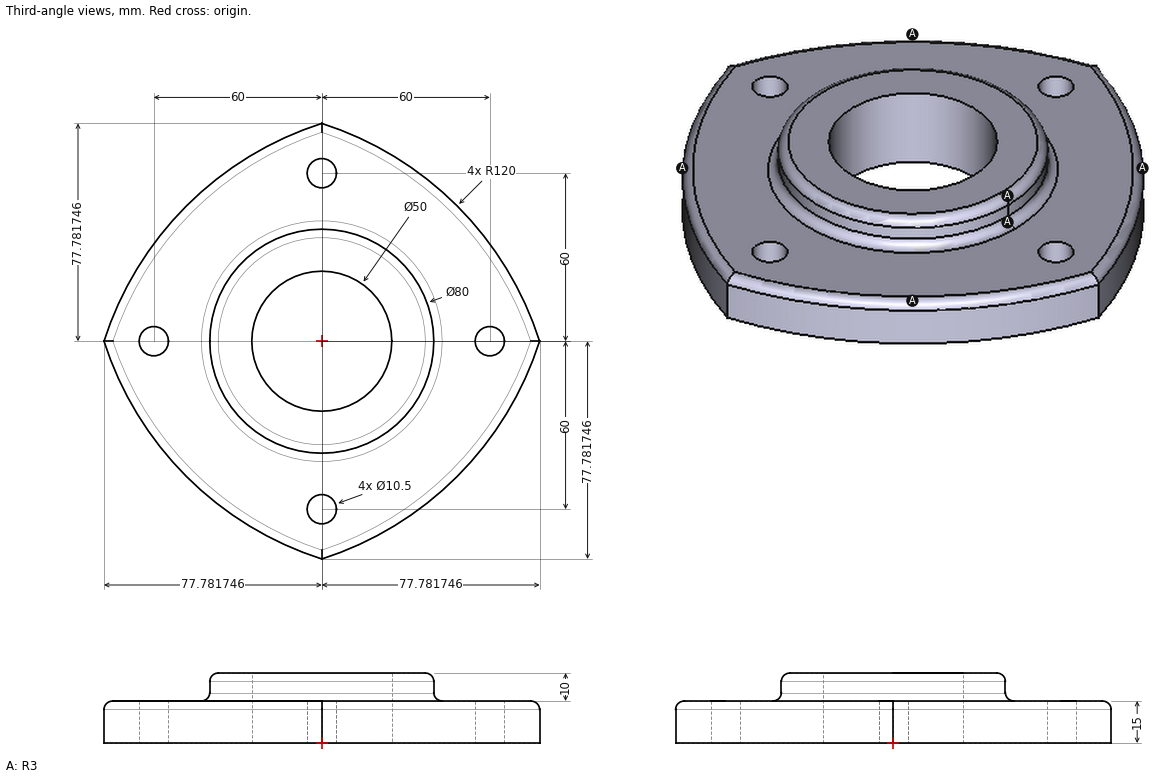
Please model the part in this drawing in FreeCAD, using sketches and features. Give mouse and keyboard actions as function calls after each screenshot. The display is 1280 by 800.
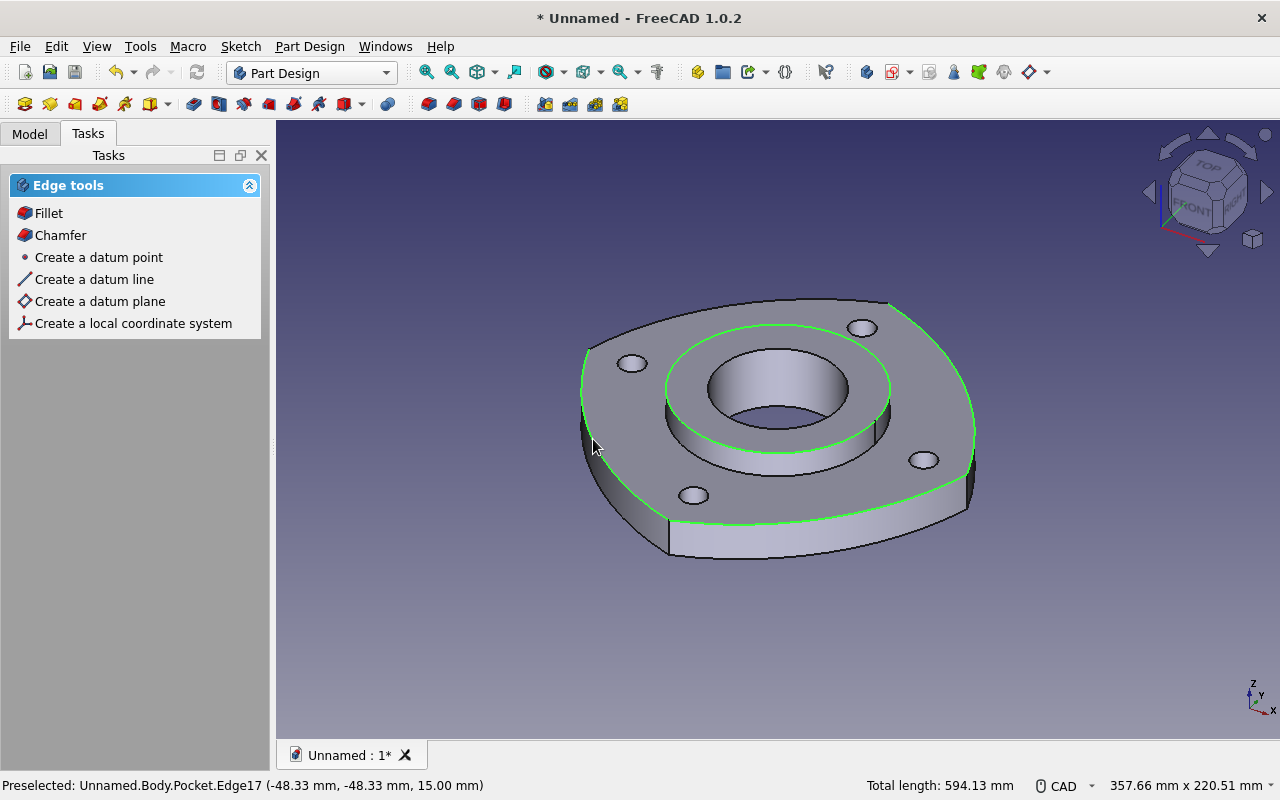
key(0)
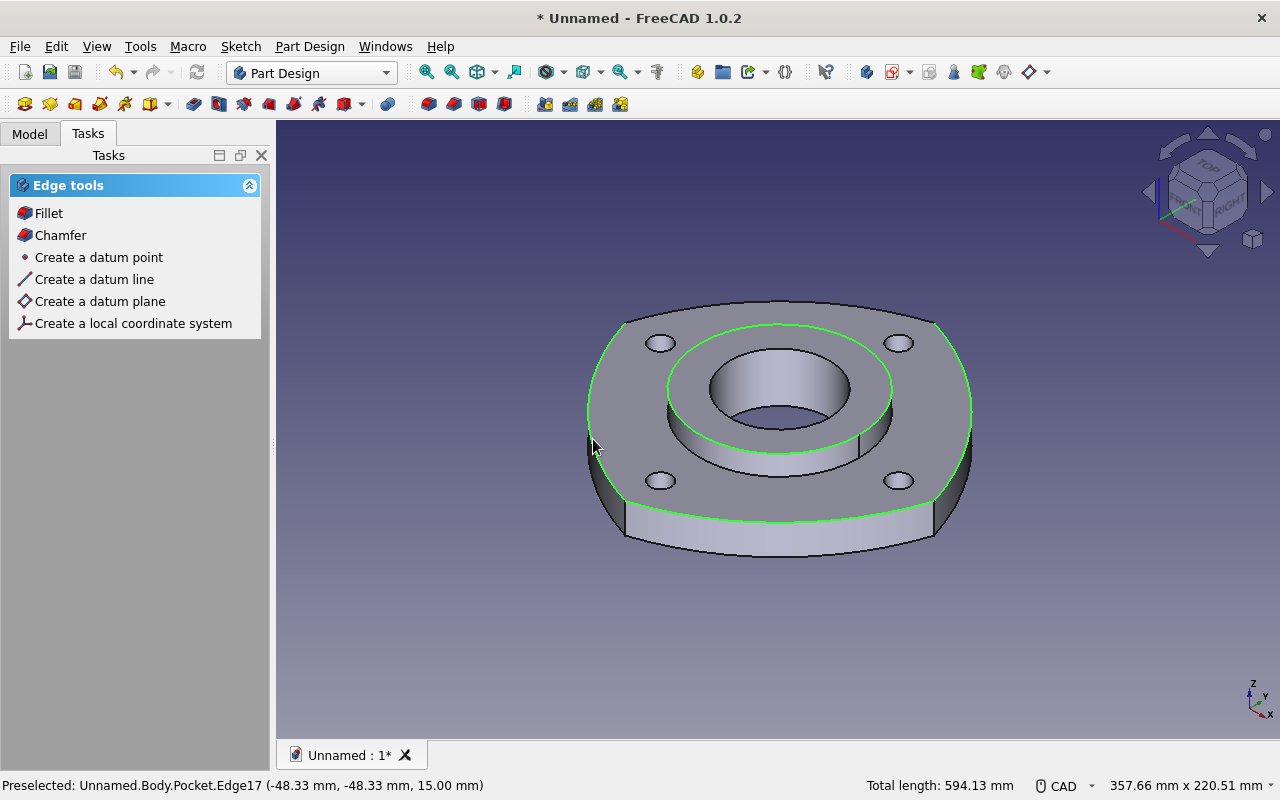
key(2)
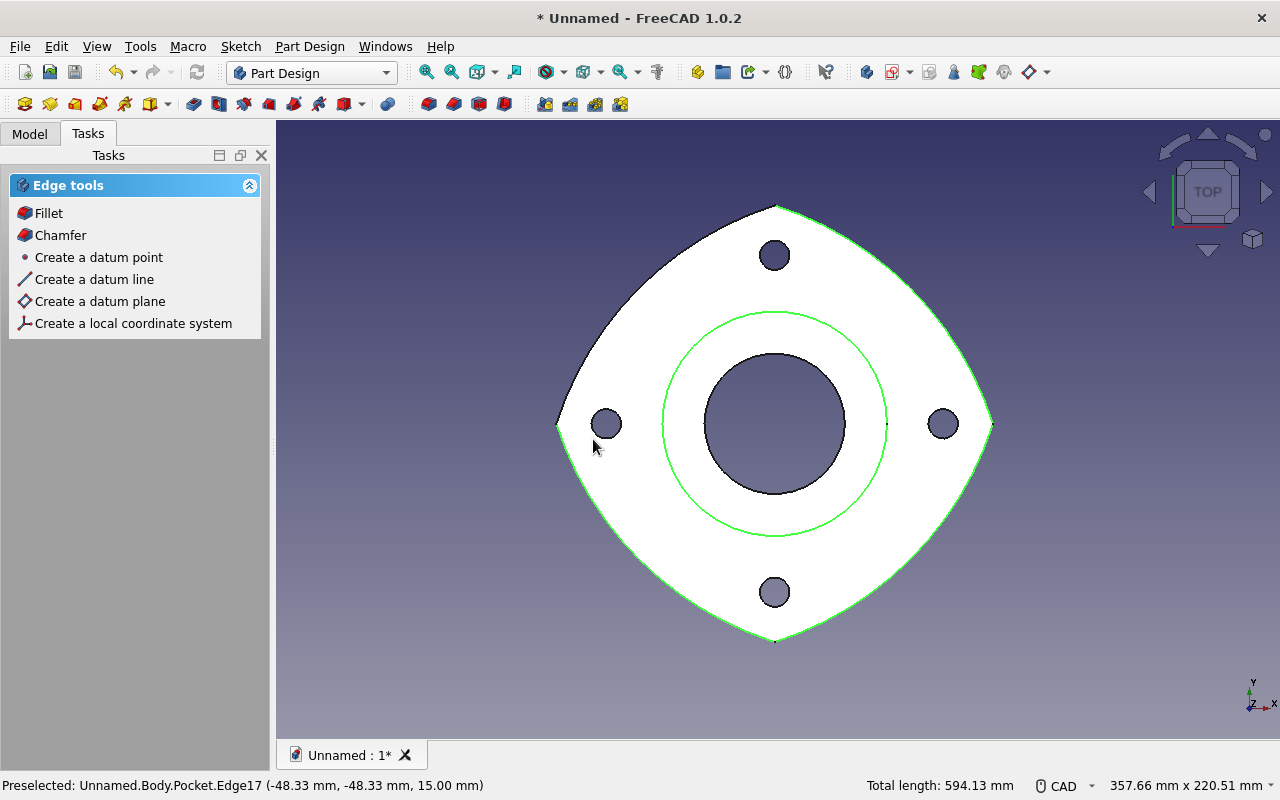
click(639, 287, ctrl)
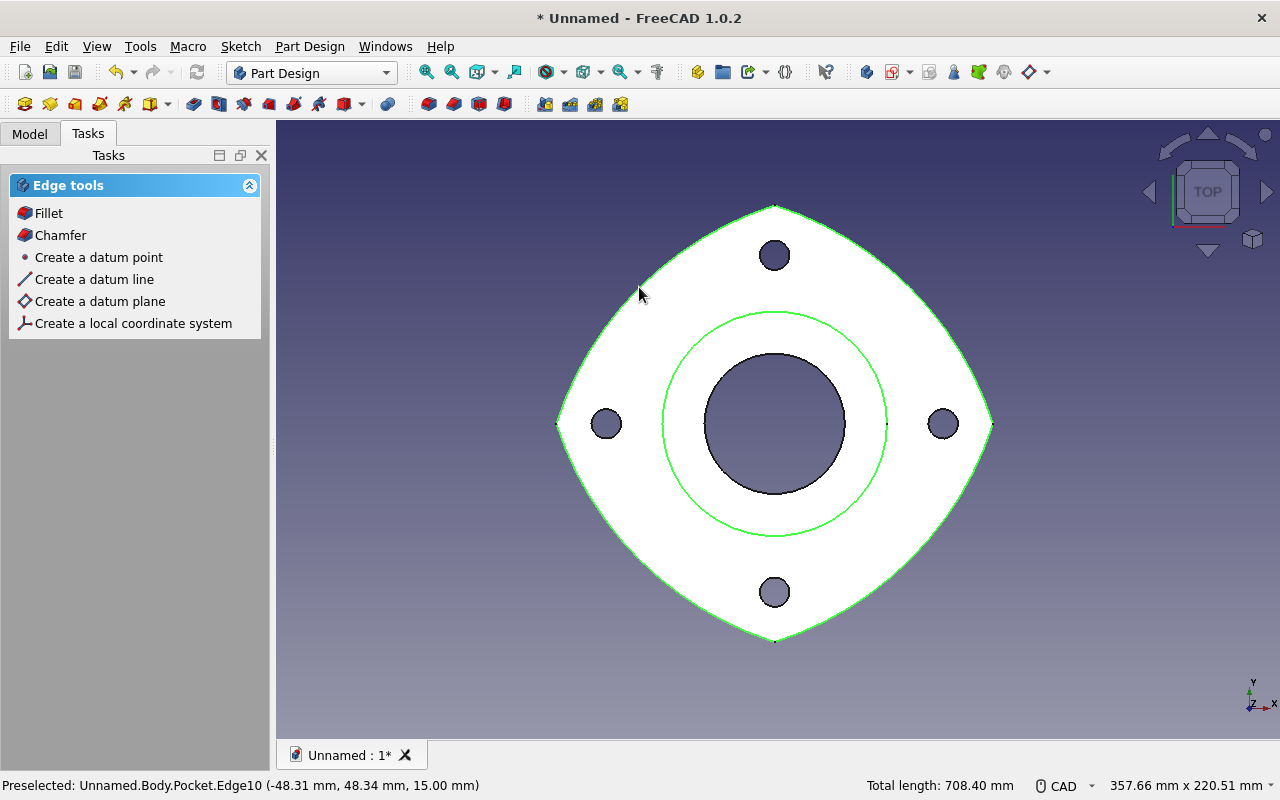
key(1)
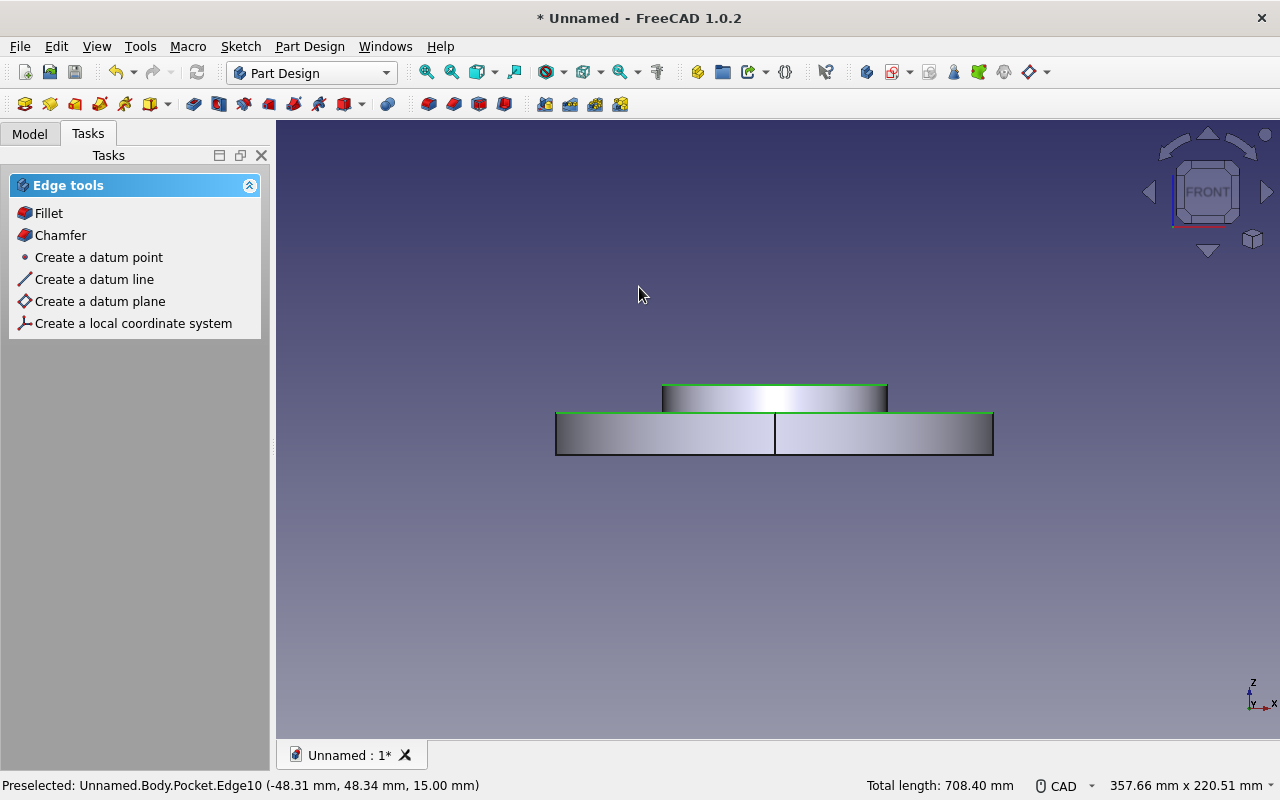
key(v)
key(f)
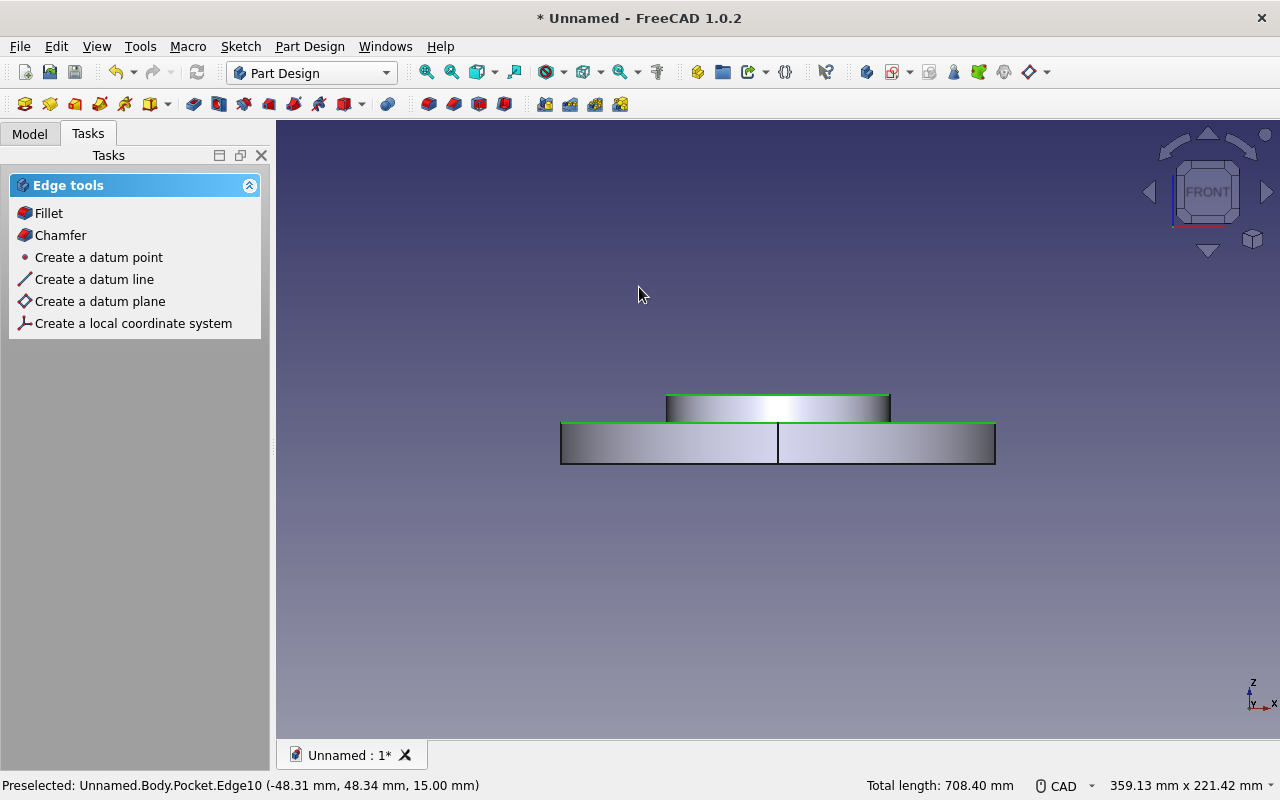
key(3)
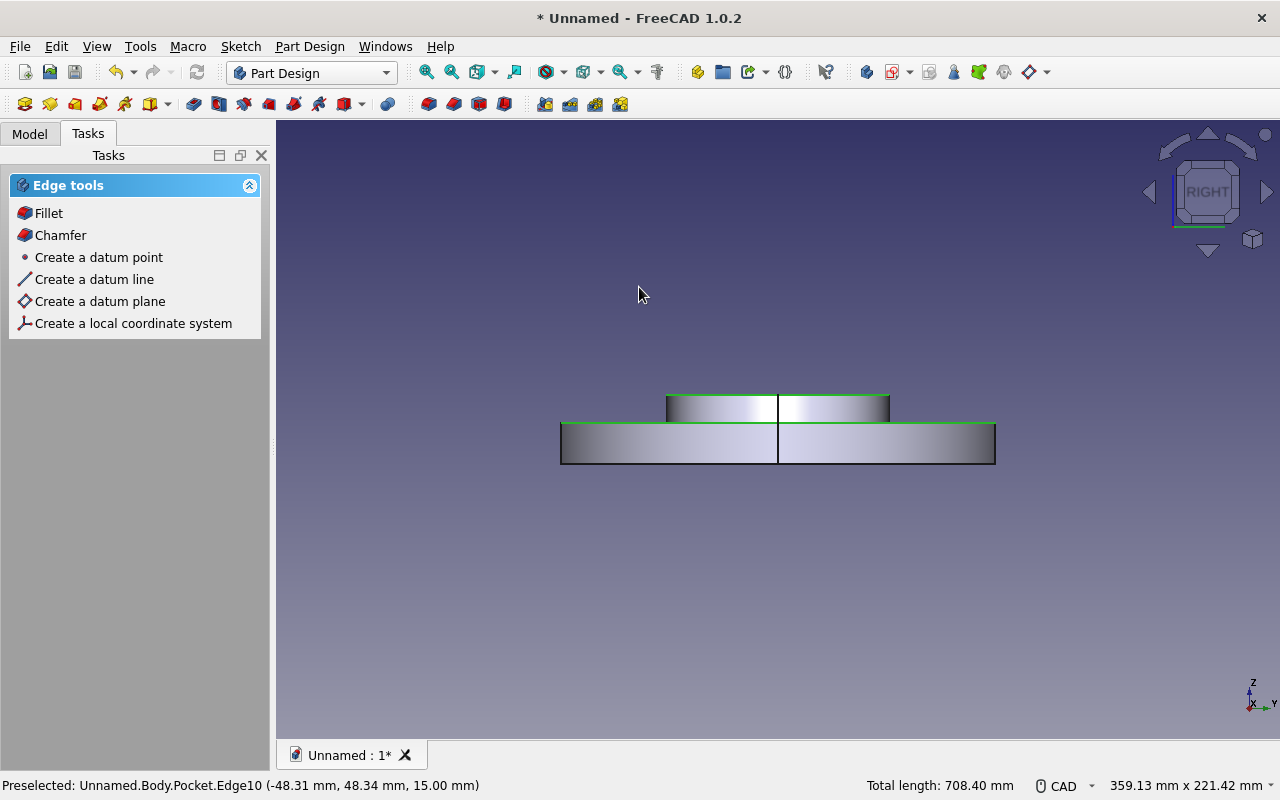
key(v)
key(f)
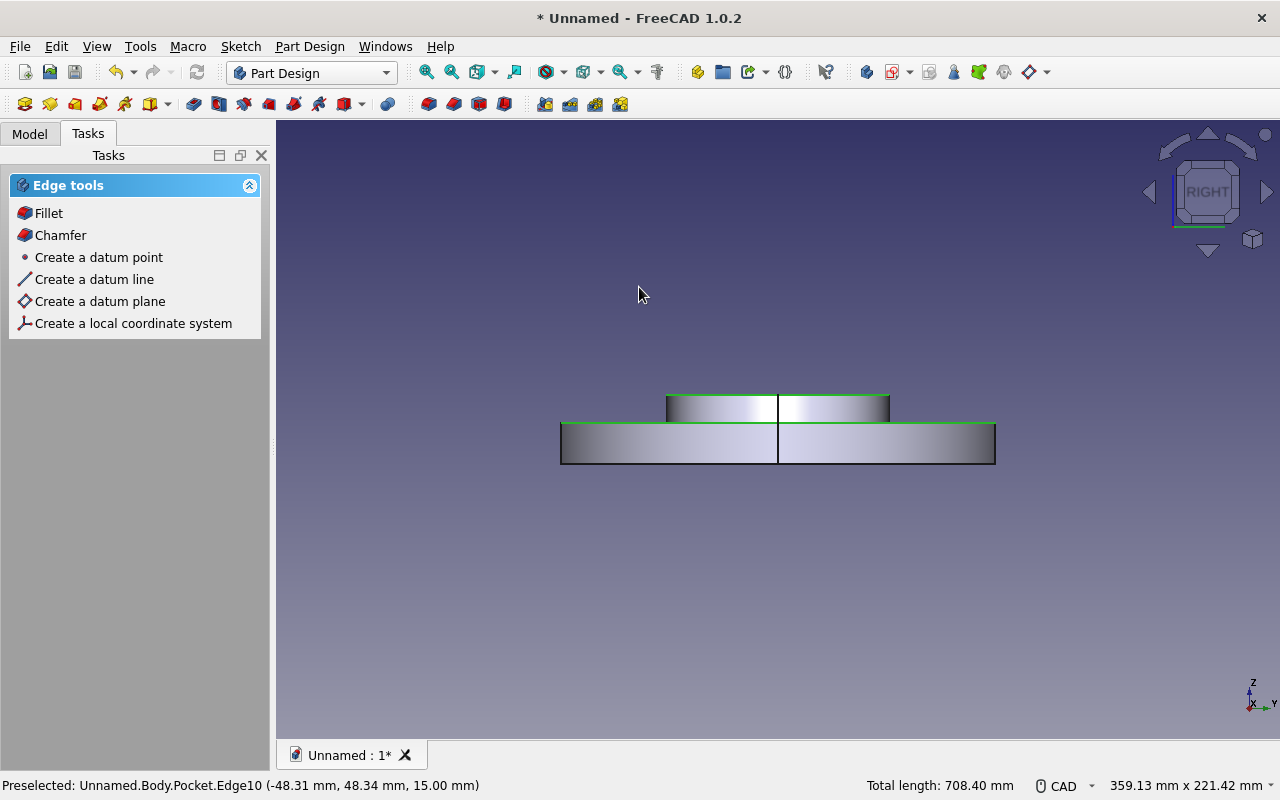
key(5)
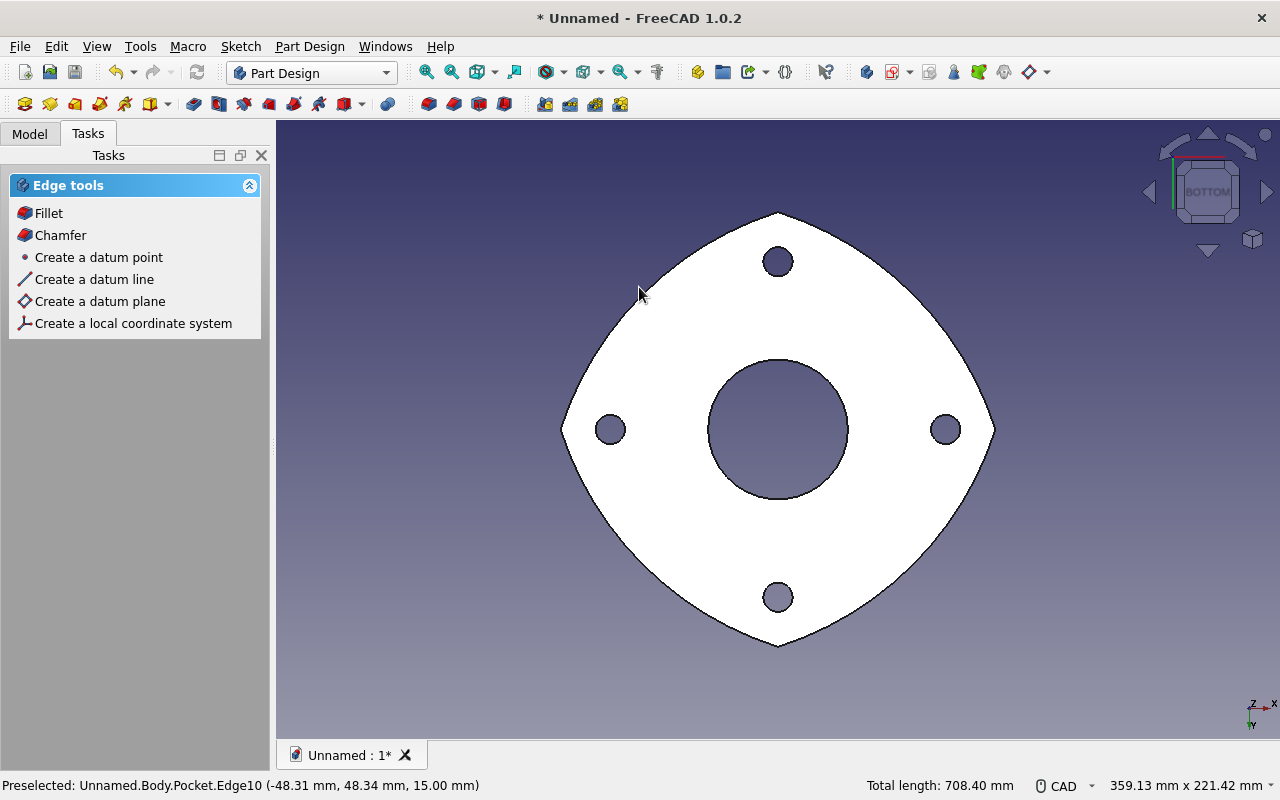
key(4)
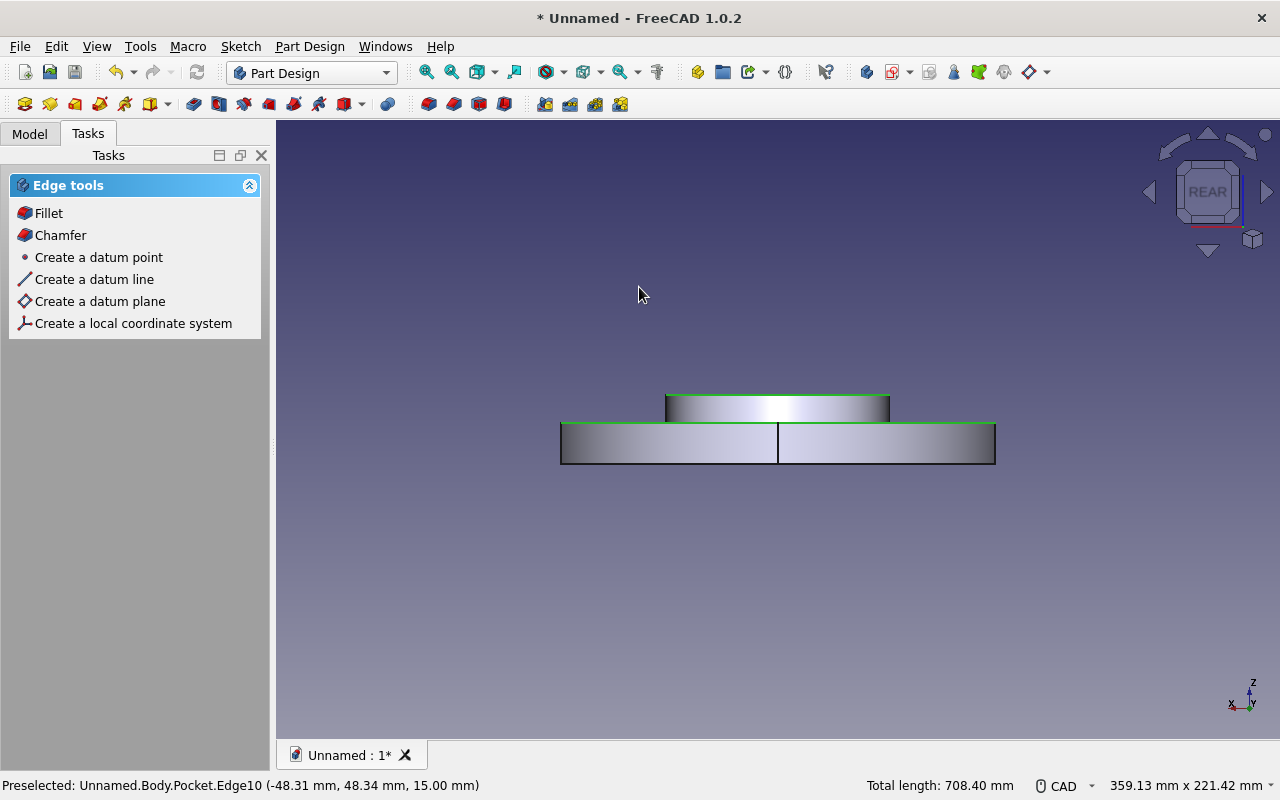
key(v)
key(f)